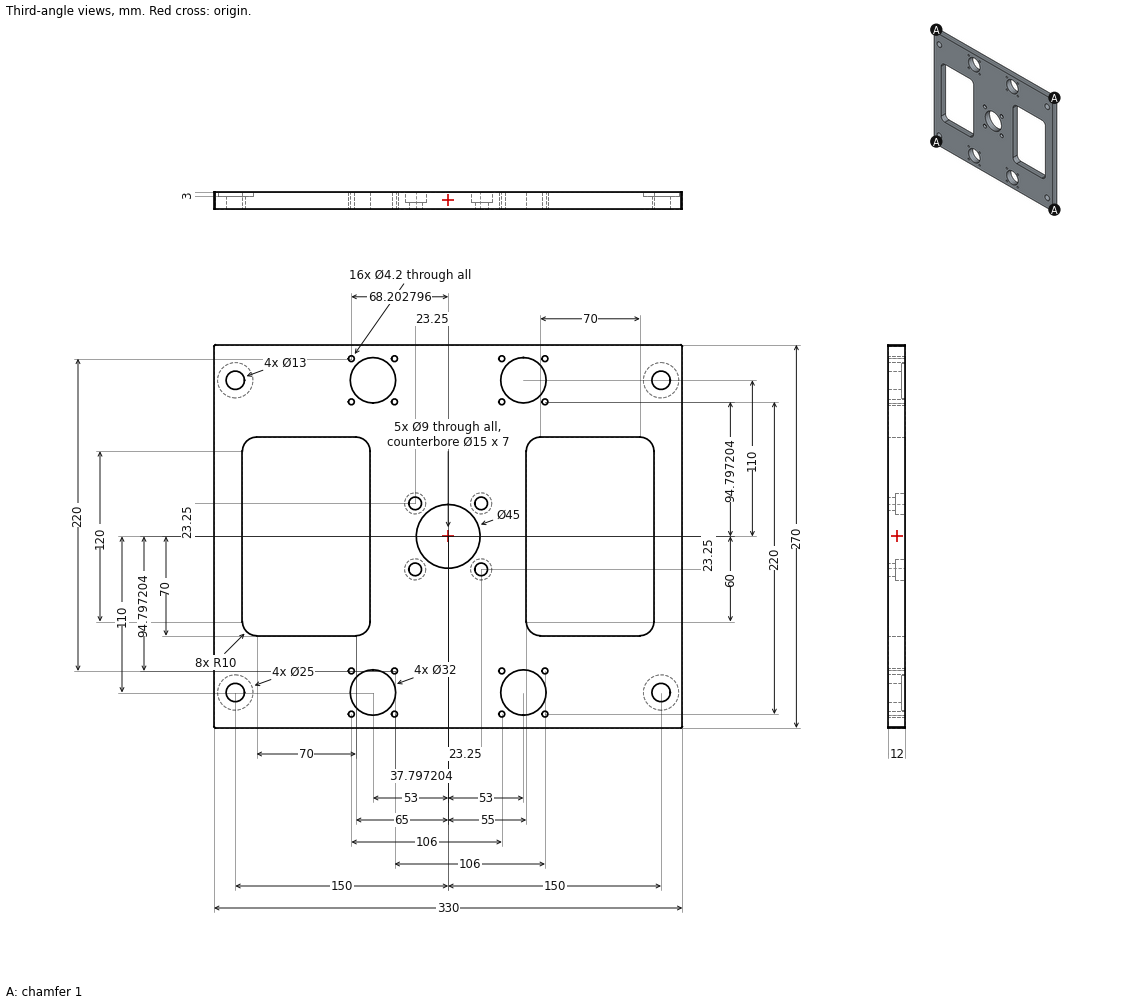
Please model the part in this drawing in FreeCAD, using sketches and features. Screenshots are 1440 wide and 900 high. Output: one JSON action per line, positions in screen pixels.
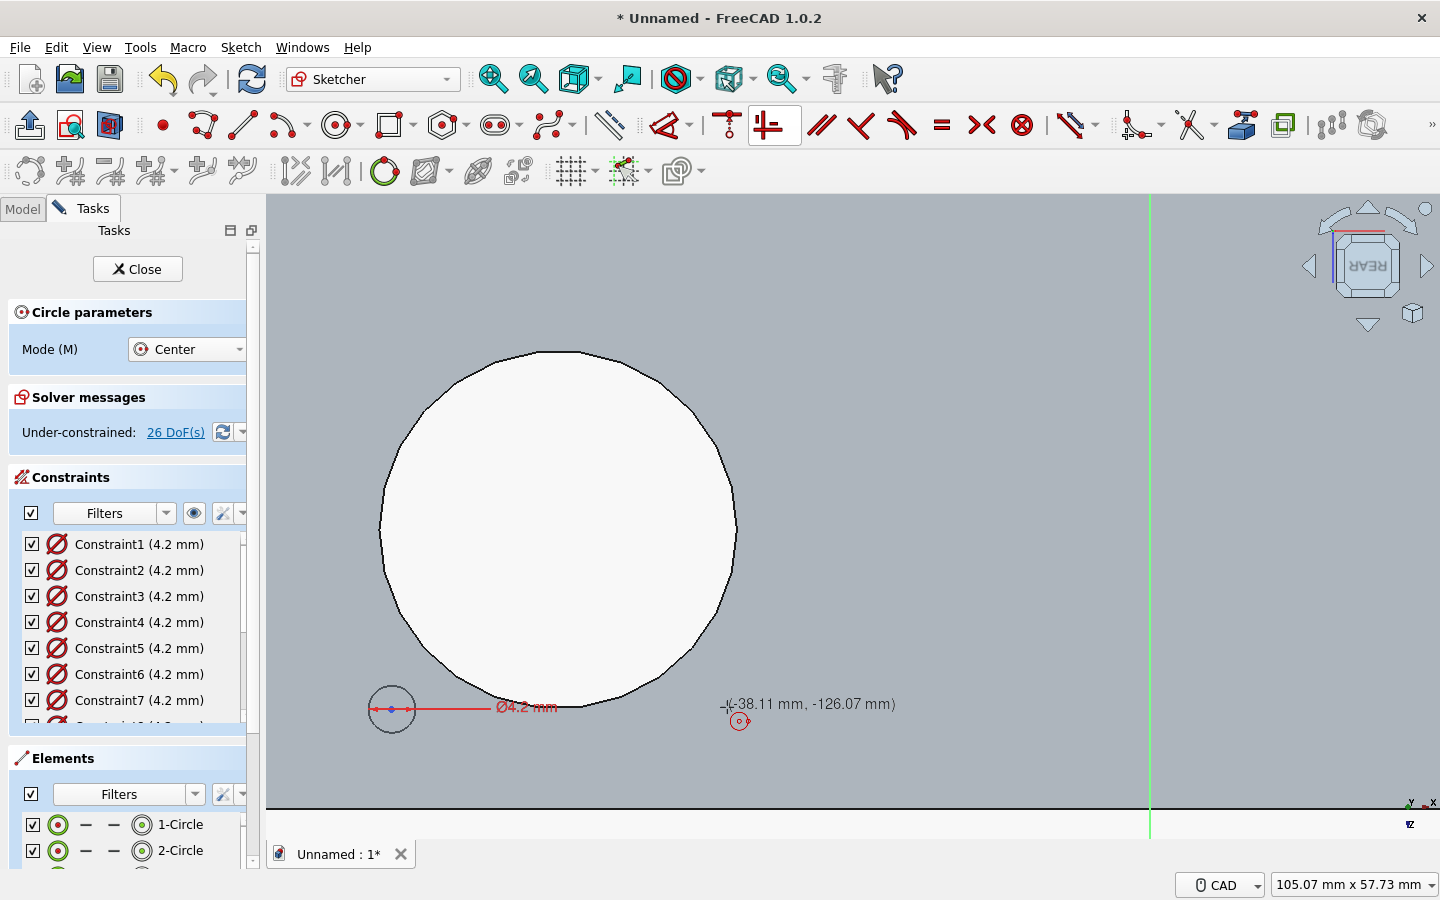
{"action": "scroll", "coordinate": [727, 707], "scroll_direction": "down", "scroll_amount": 10}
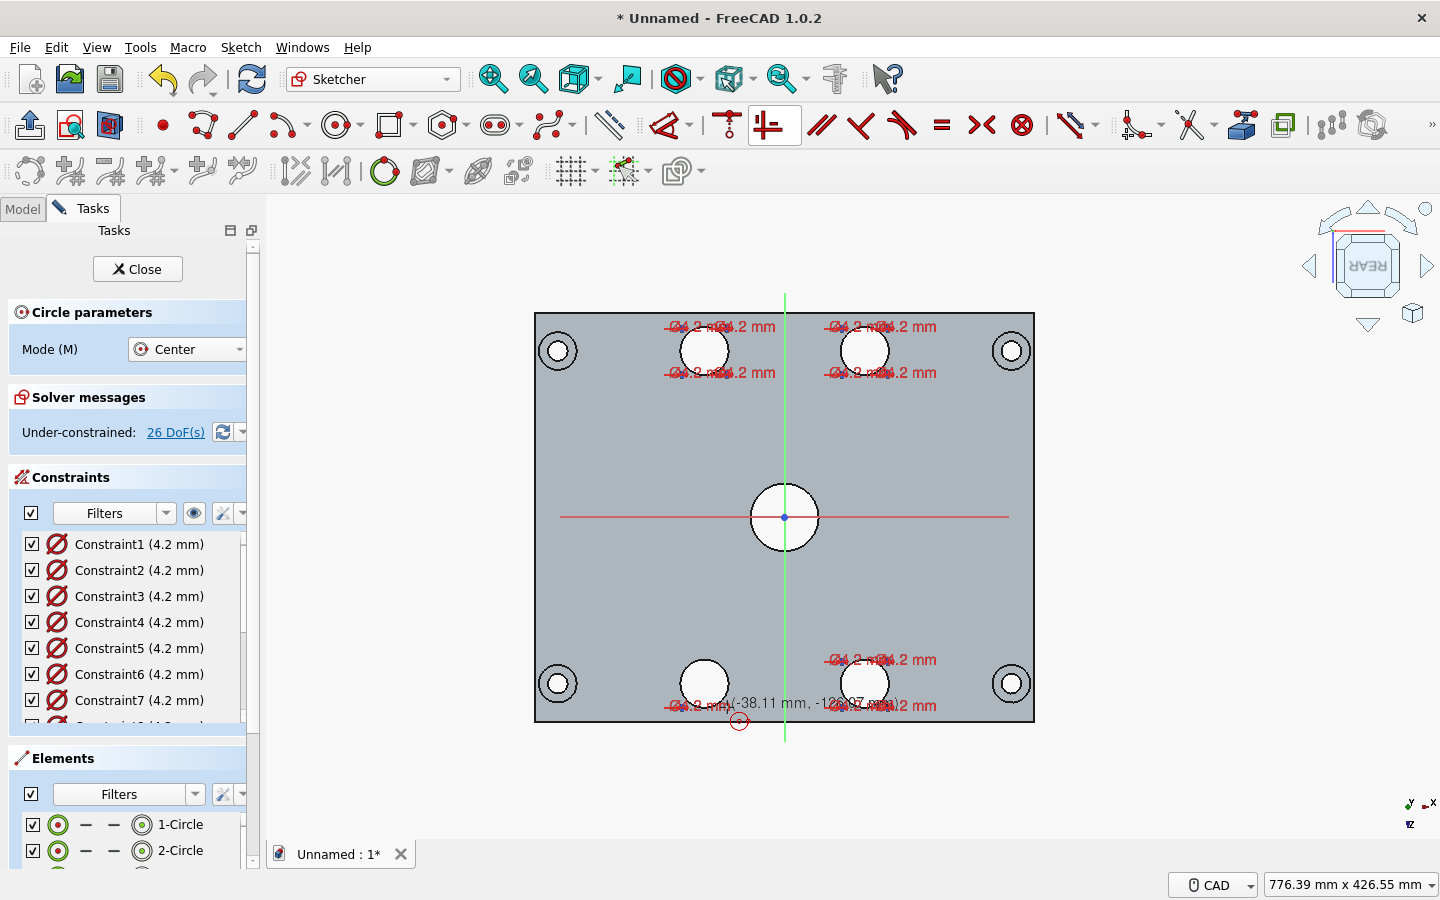
{"action": "left_click", "coordinate": [727, 707]}
{"action": "mouse_move", "coordinate": [730, 704]}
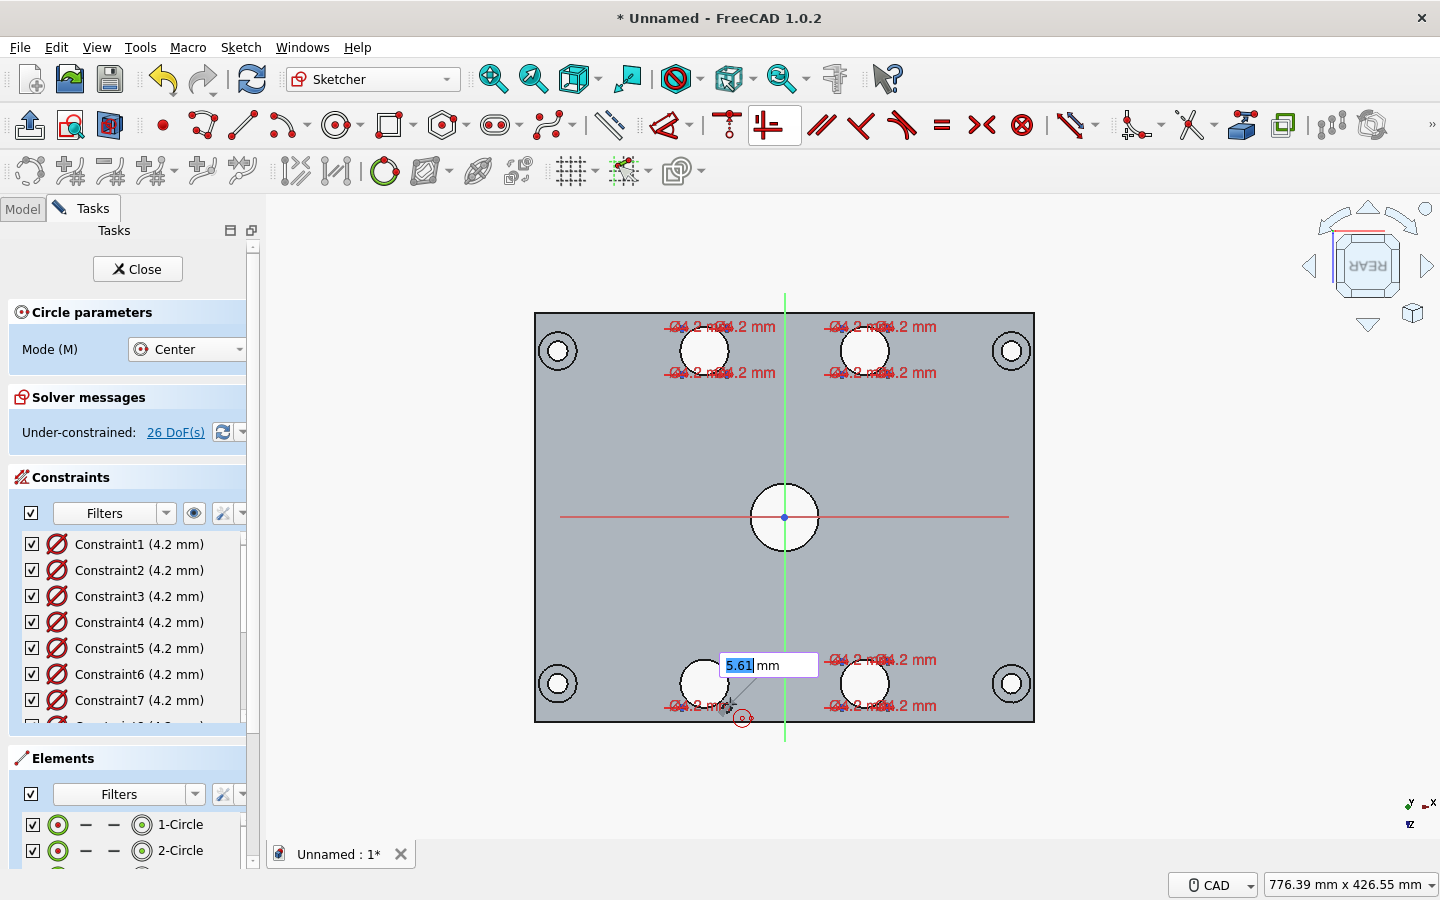
{"action": "type", "text": "4.2"}
{"action": "key", "text": "Return"}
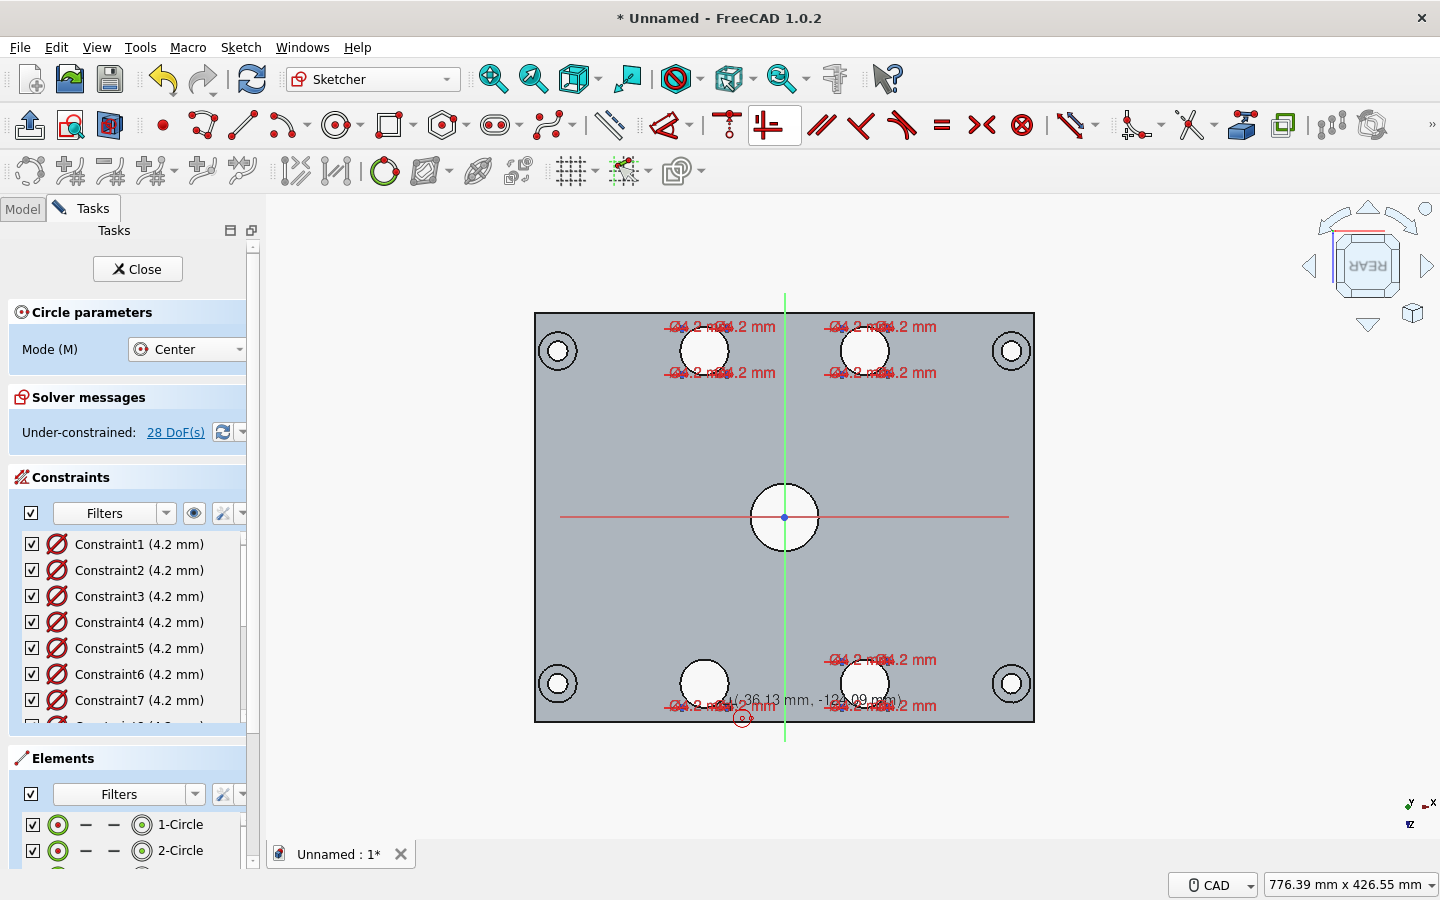
{"action": "scroll", "coordinate": [727, 661], "scroll_direction": "up", "scroll_amount": 10}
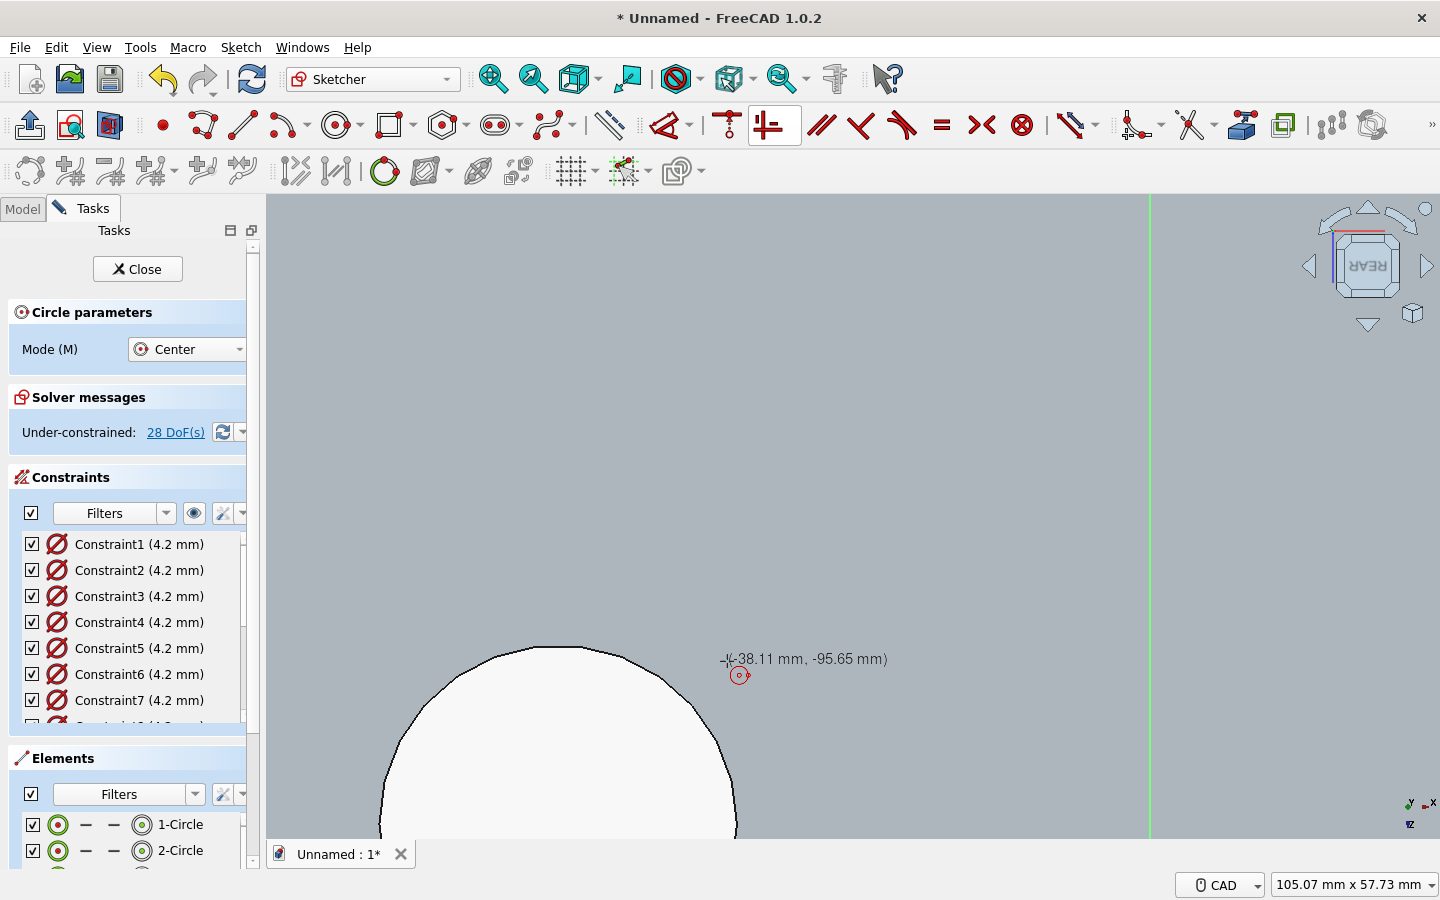
{"action": "scroll", "coordinate": [727, 661], "scroll_direction": "down", "scroll_amount": 10}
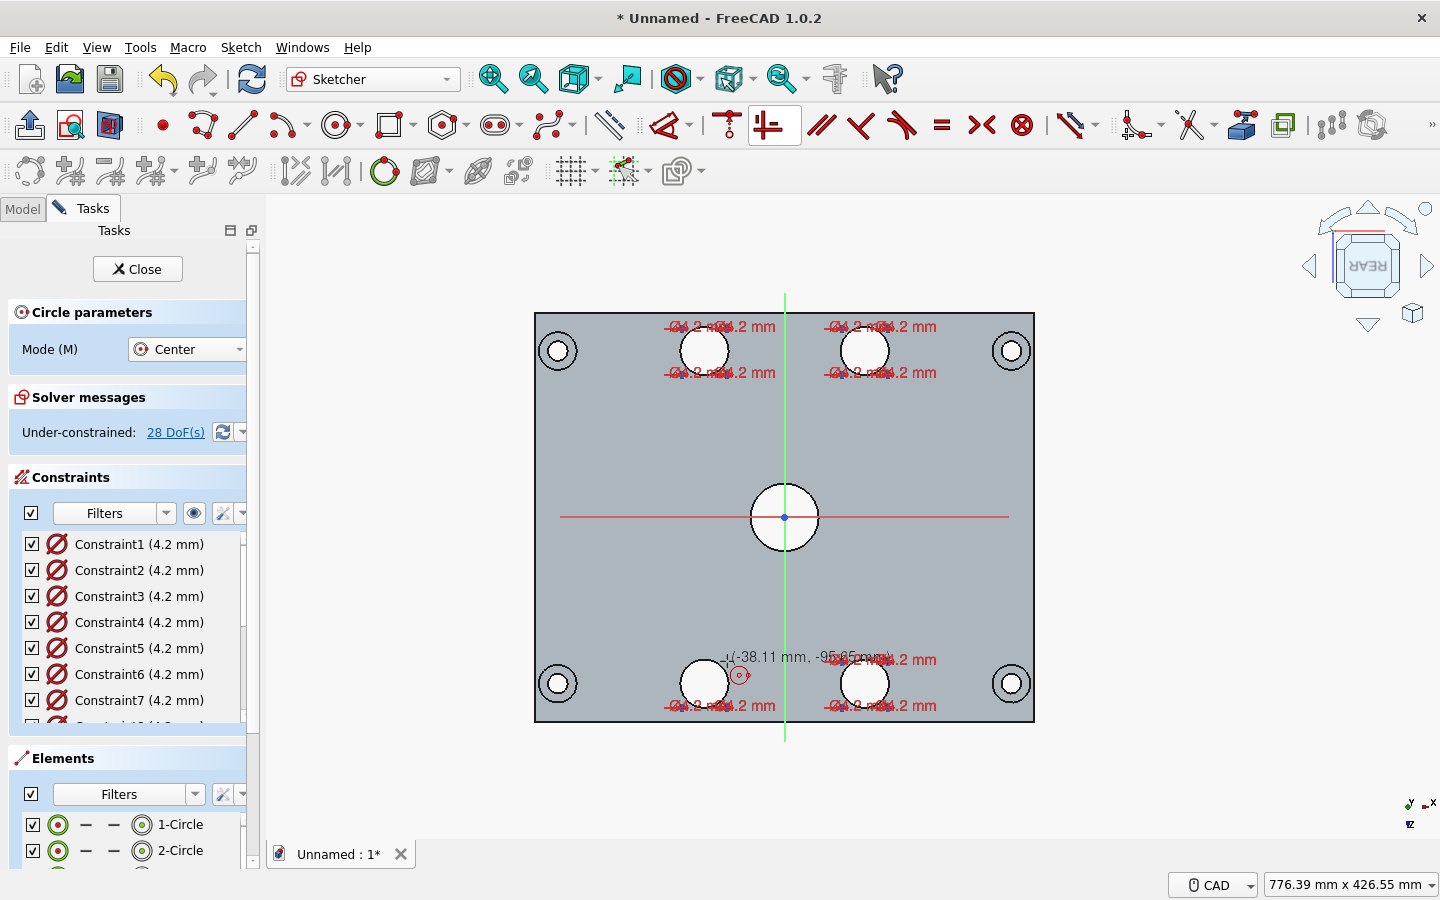
{"action": "left_click", "coordinate": [727, 661]}
{"action": "mouse_move", "coordinate": [730, 658]}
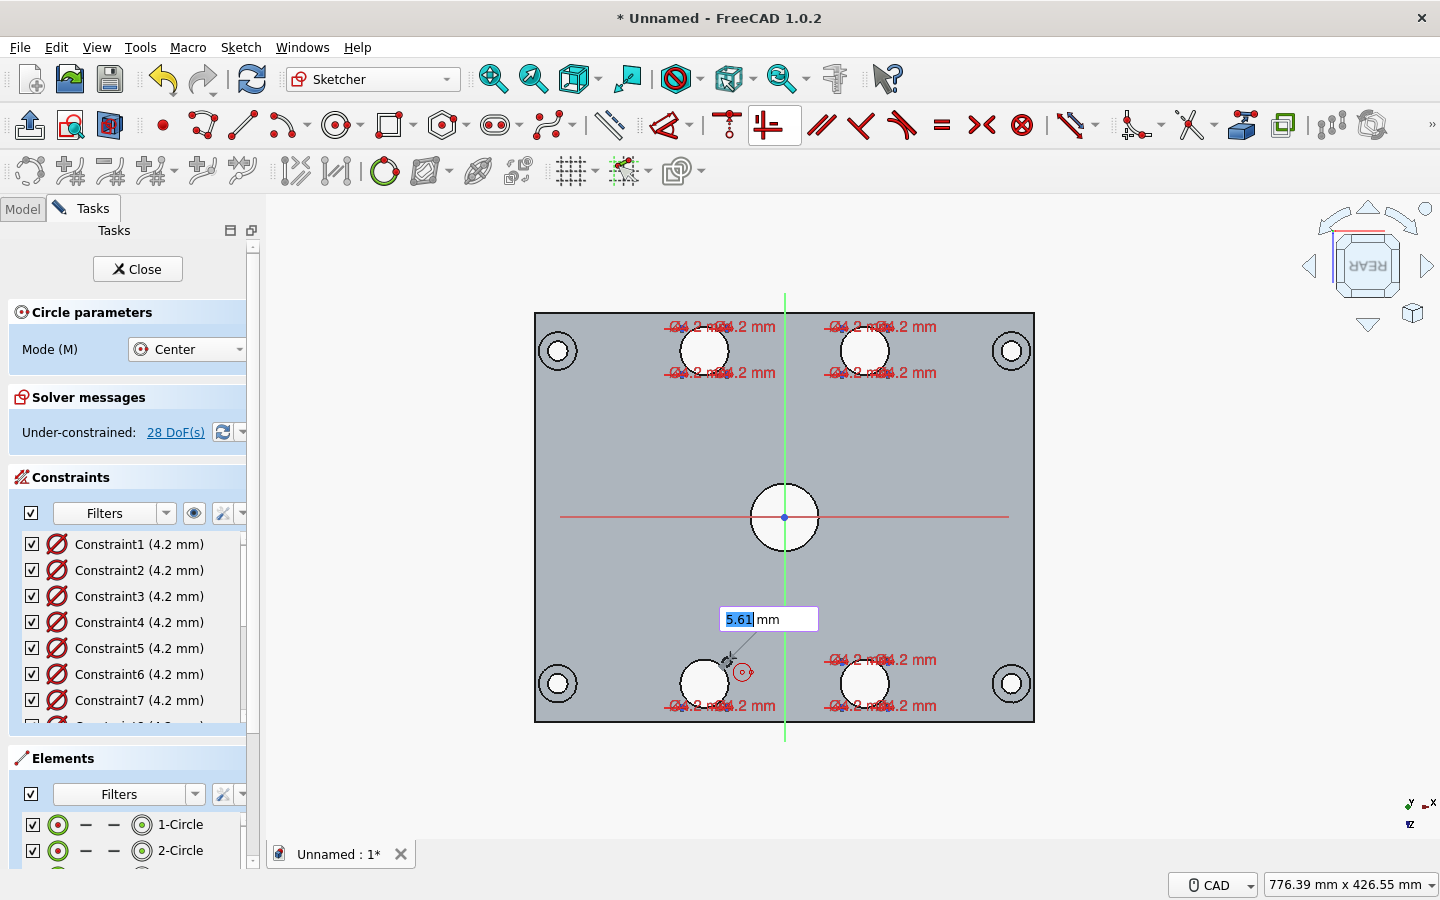
{"action": "type", "text": "4.2"}
{"action": "key", "text": "Return"}